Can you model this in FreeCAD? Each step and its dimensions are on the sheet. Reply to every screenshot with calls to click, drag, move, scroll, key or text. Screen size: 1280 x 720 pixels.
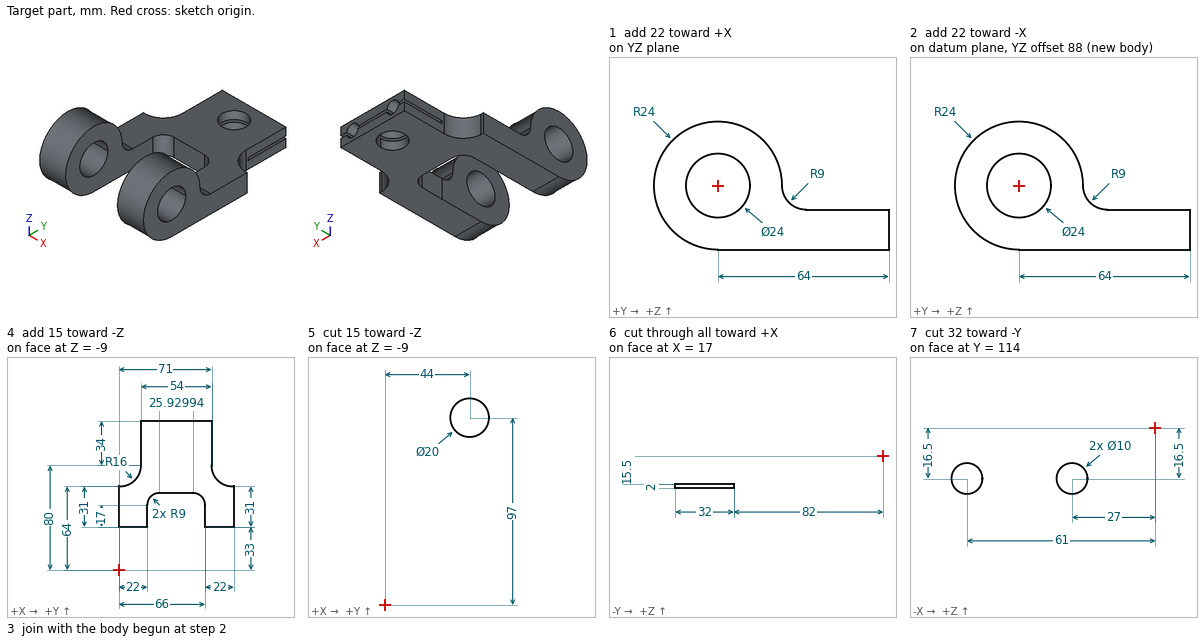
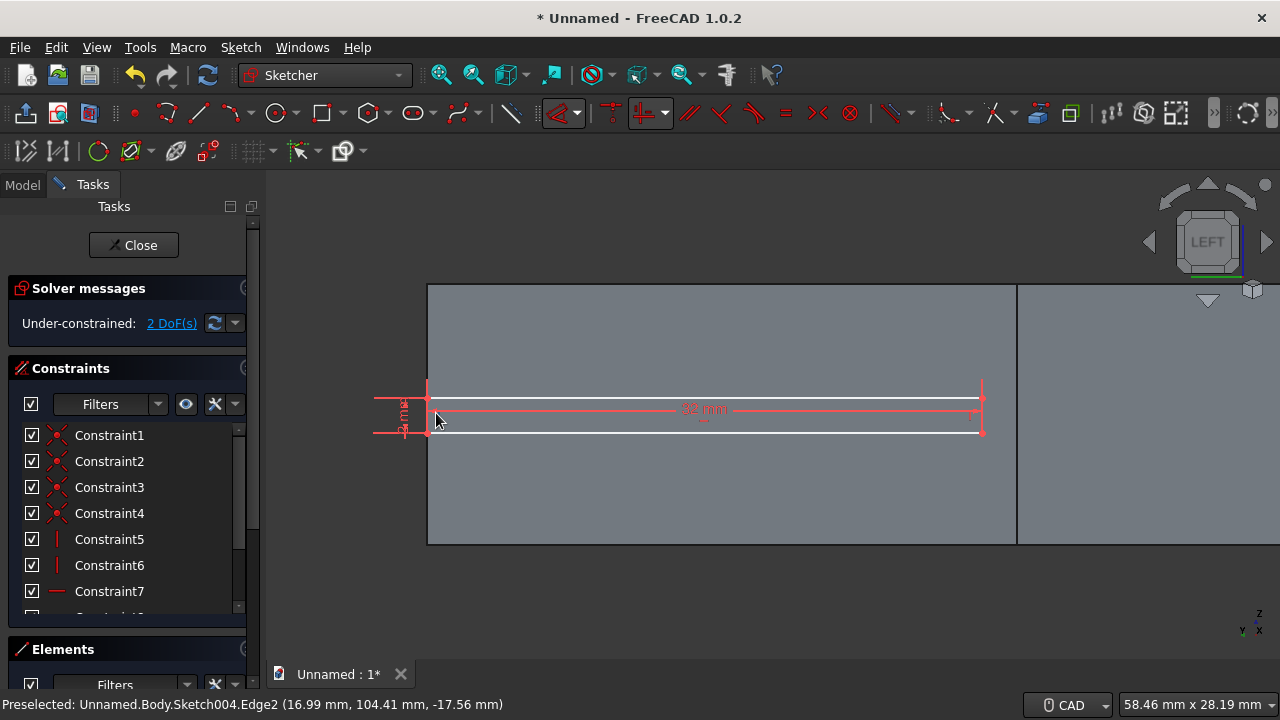
click(982, 433)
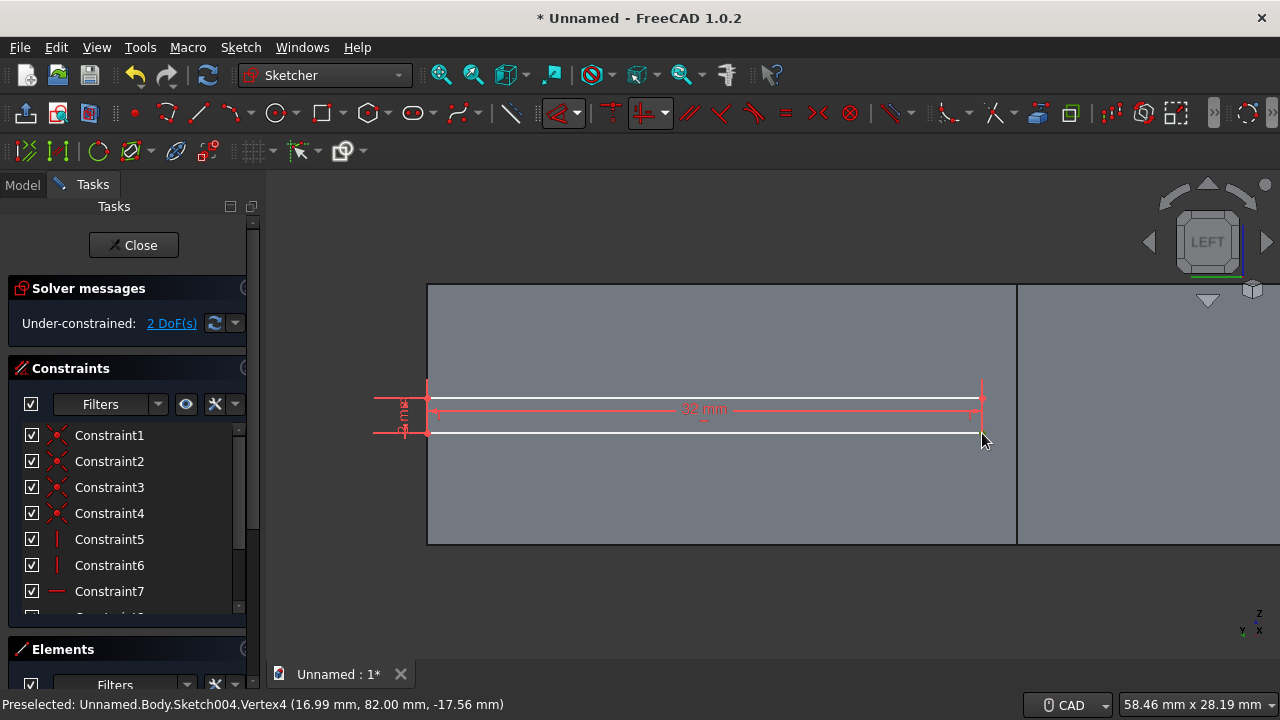
key(l)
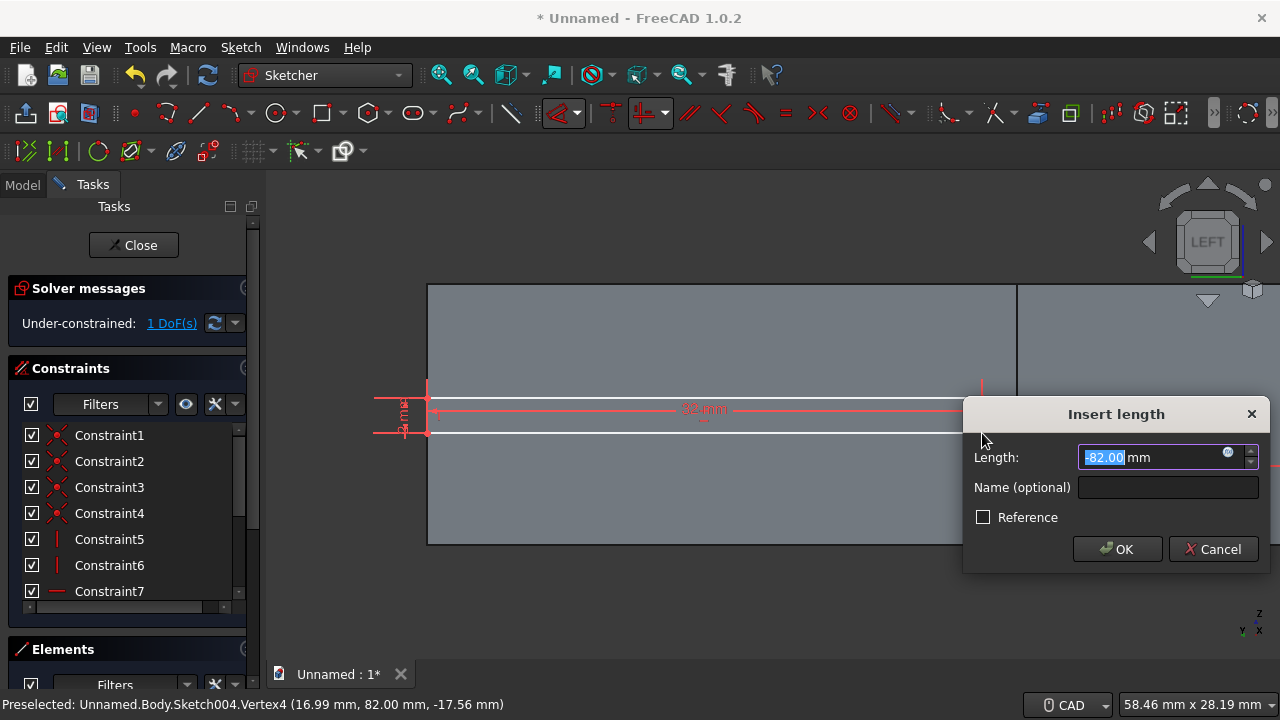
text(-82)
key(Return)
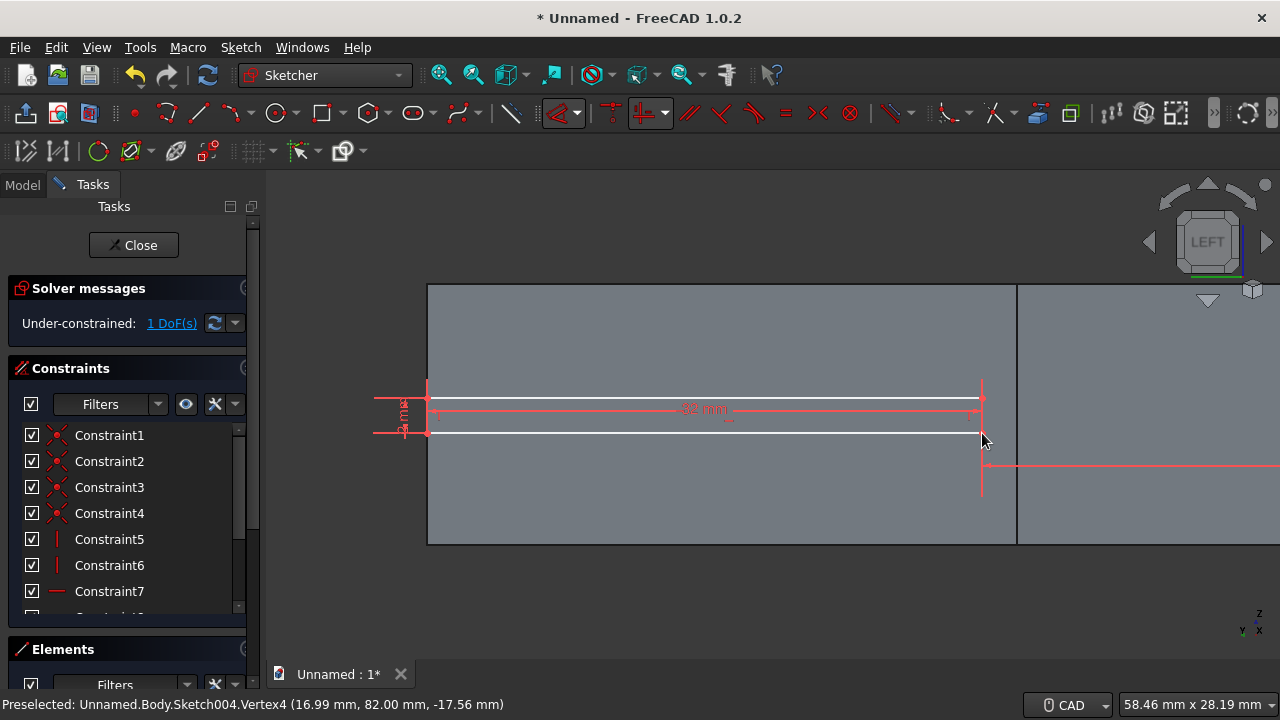
click(427, 398)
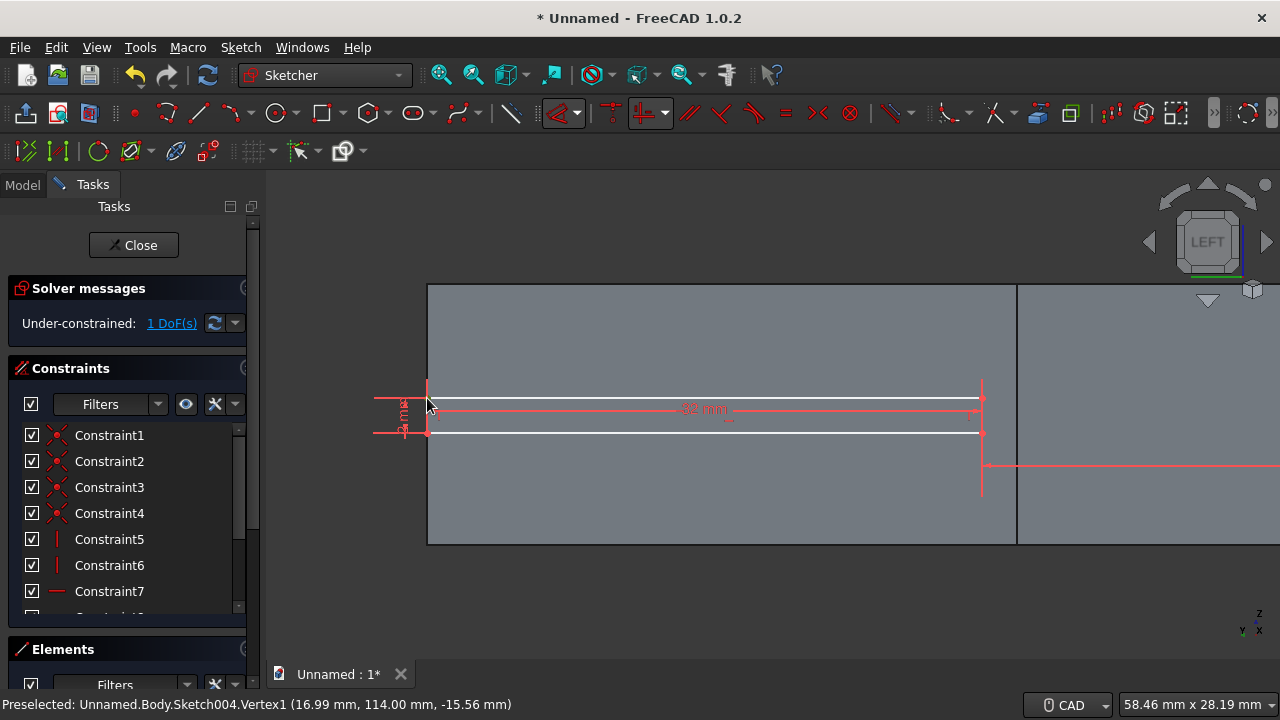
click(580, 114)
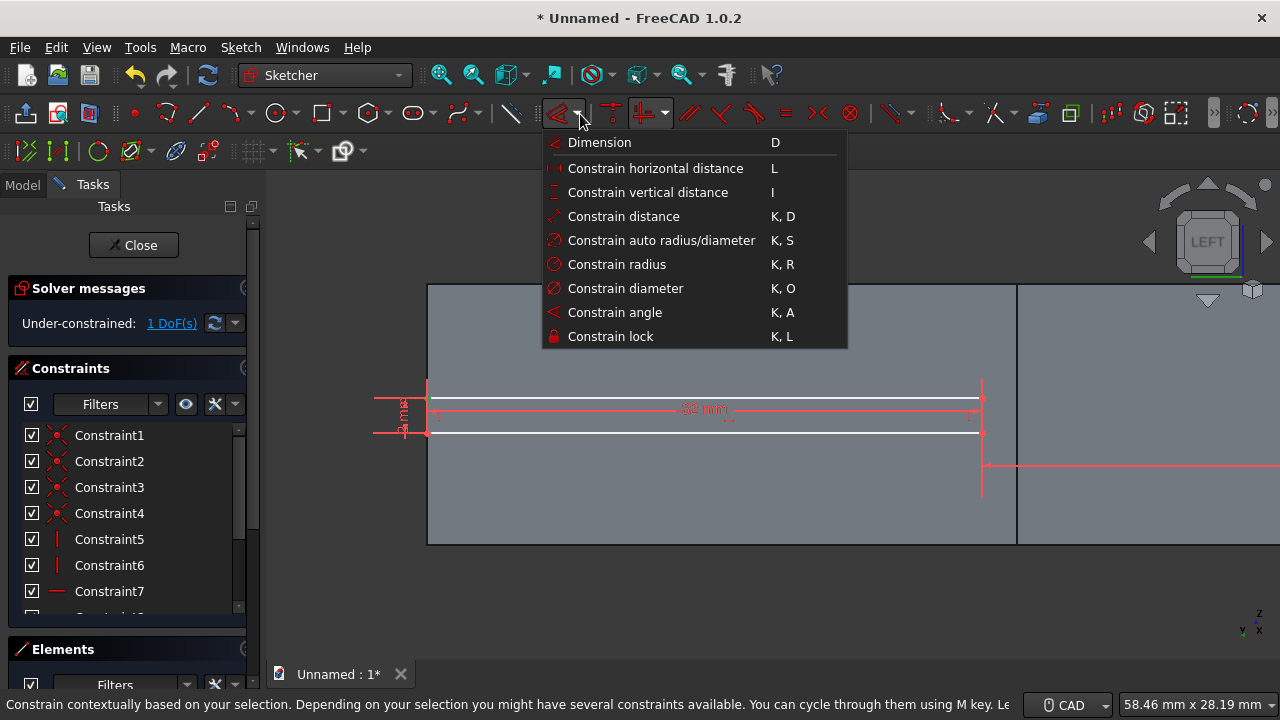
click(695, 192)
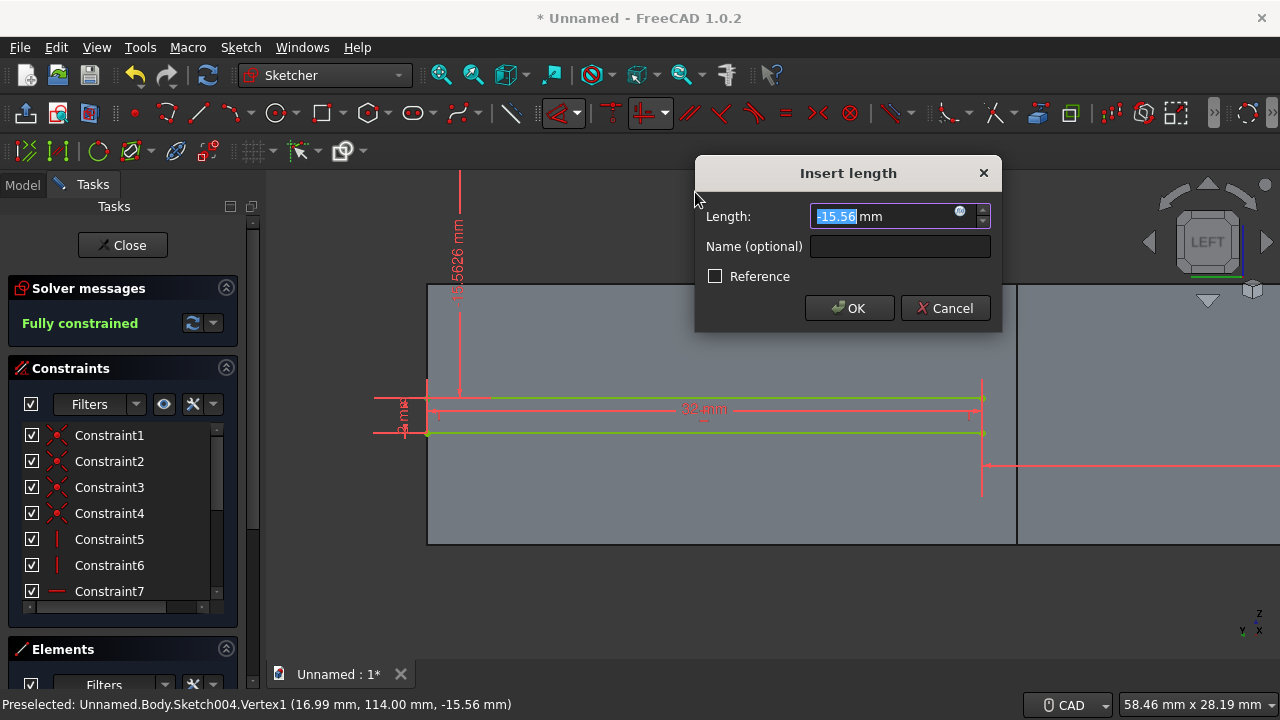
text(-15.5)
key(Return)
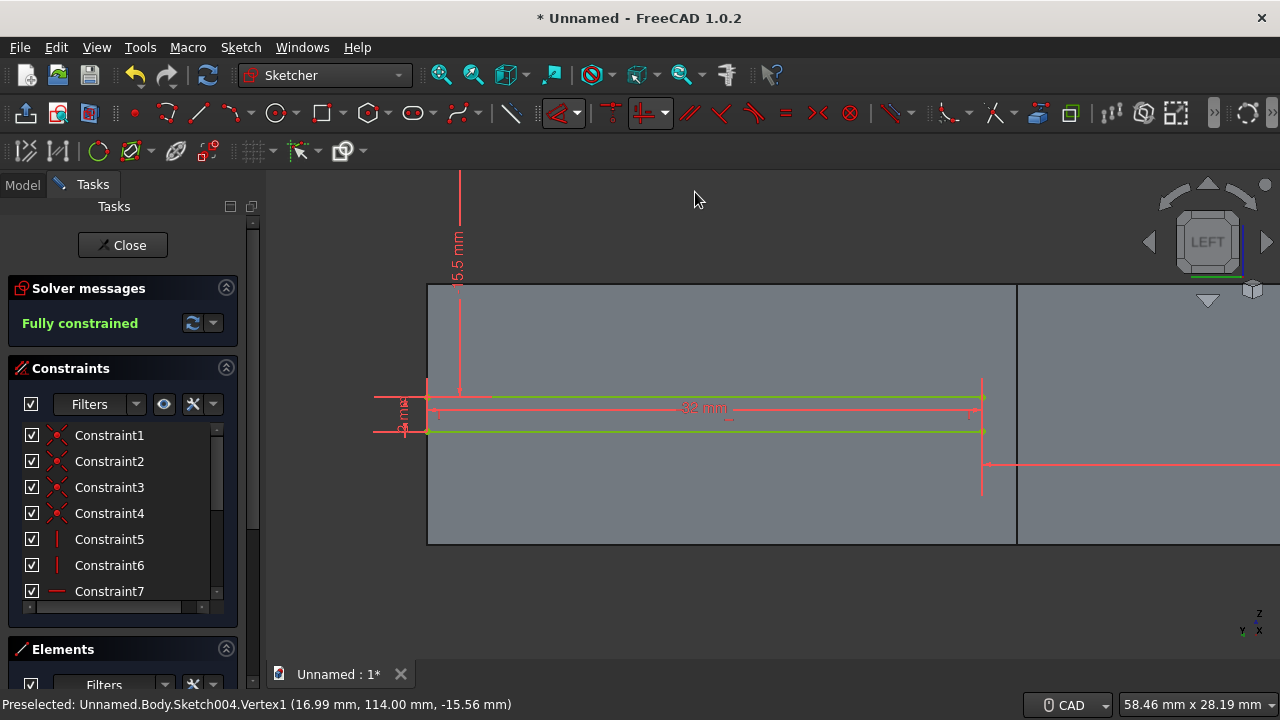
click(123, 245)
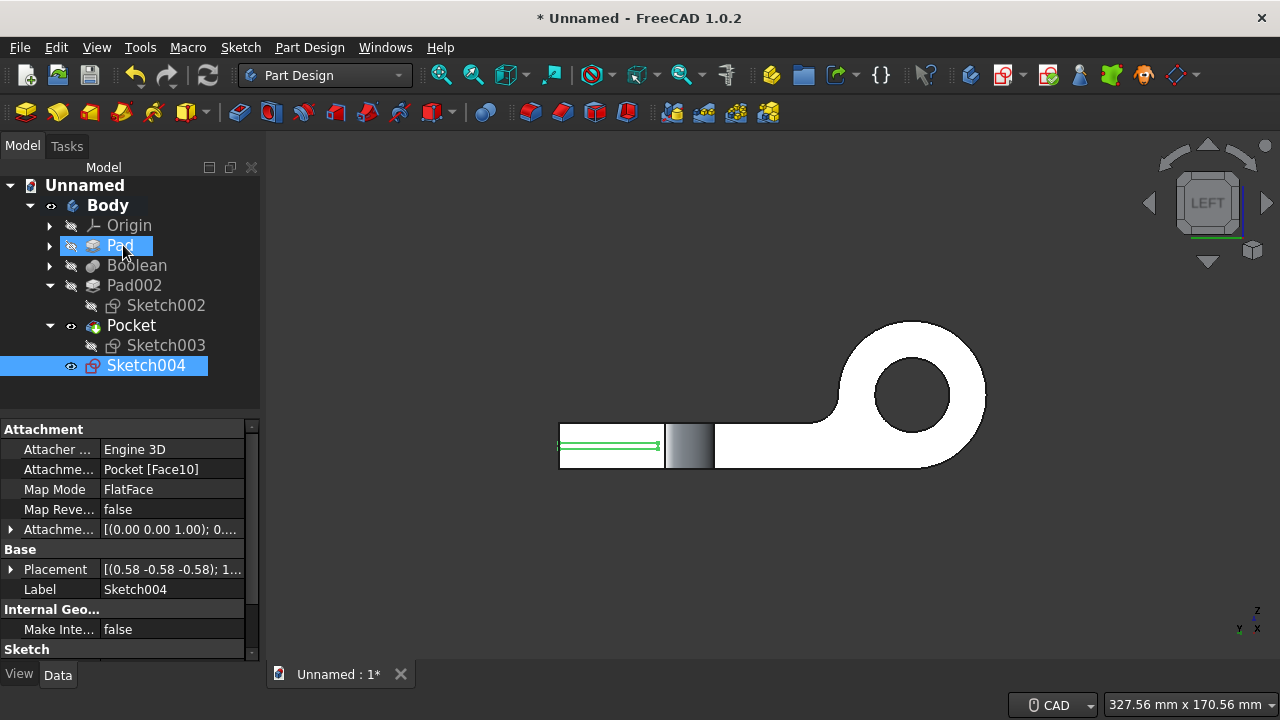
click(240, 112)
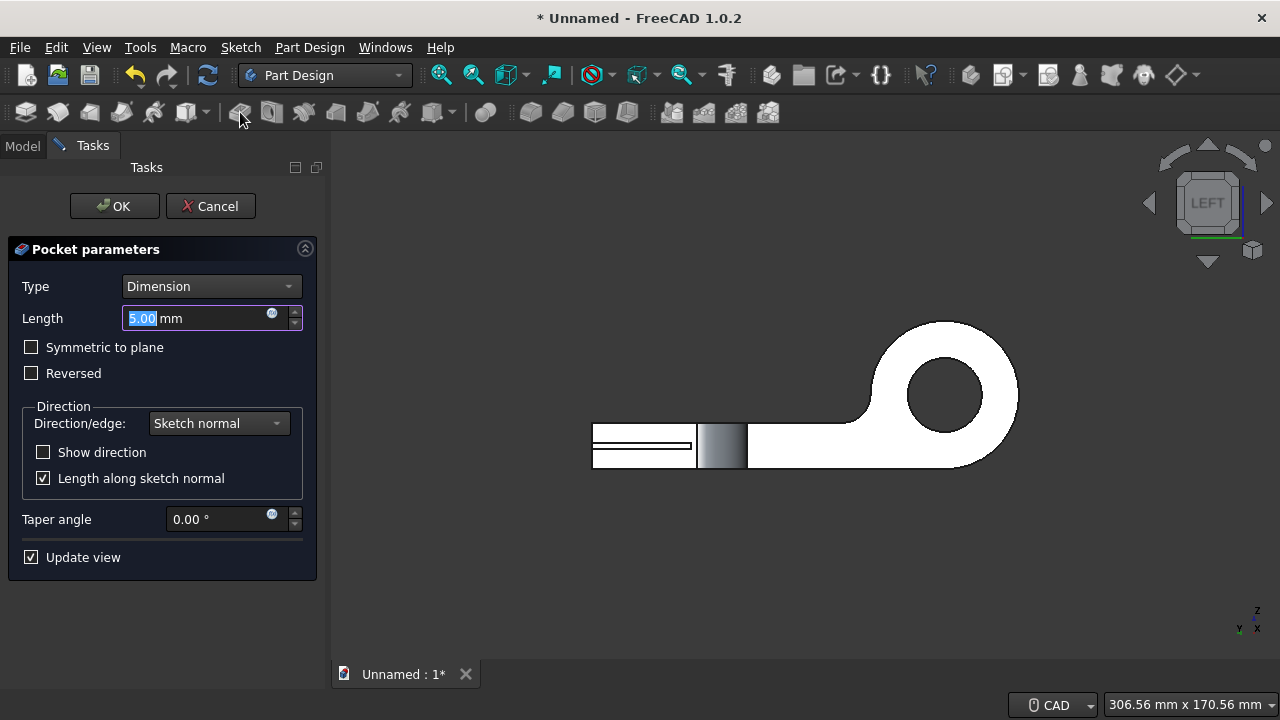
click(212, 286)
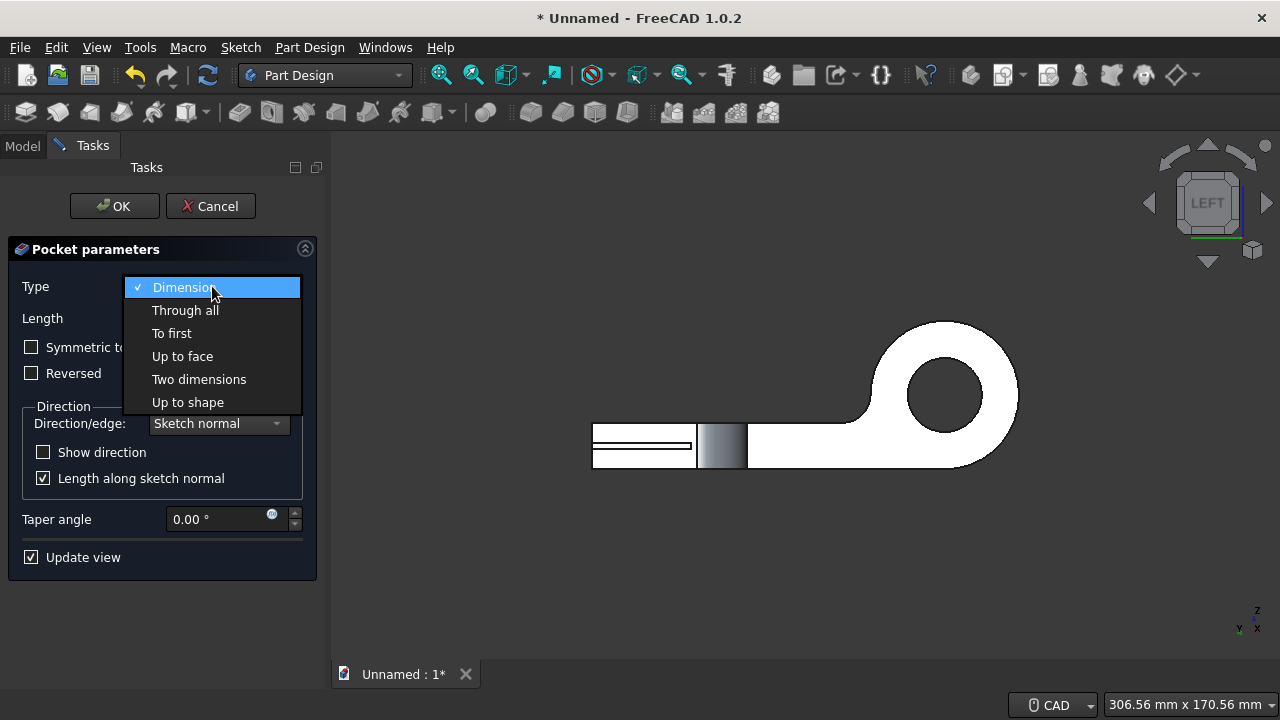
click(212, 310)